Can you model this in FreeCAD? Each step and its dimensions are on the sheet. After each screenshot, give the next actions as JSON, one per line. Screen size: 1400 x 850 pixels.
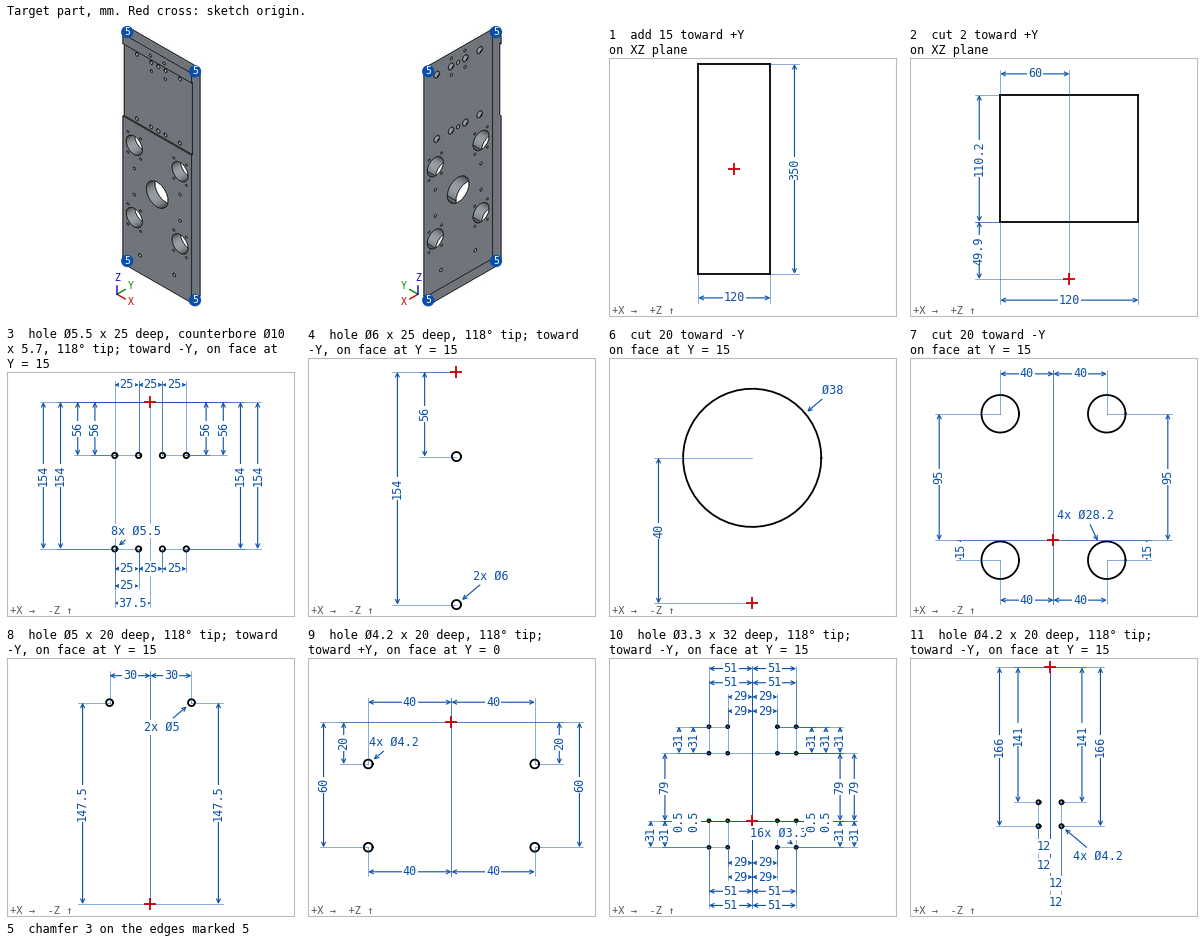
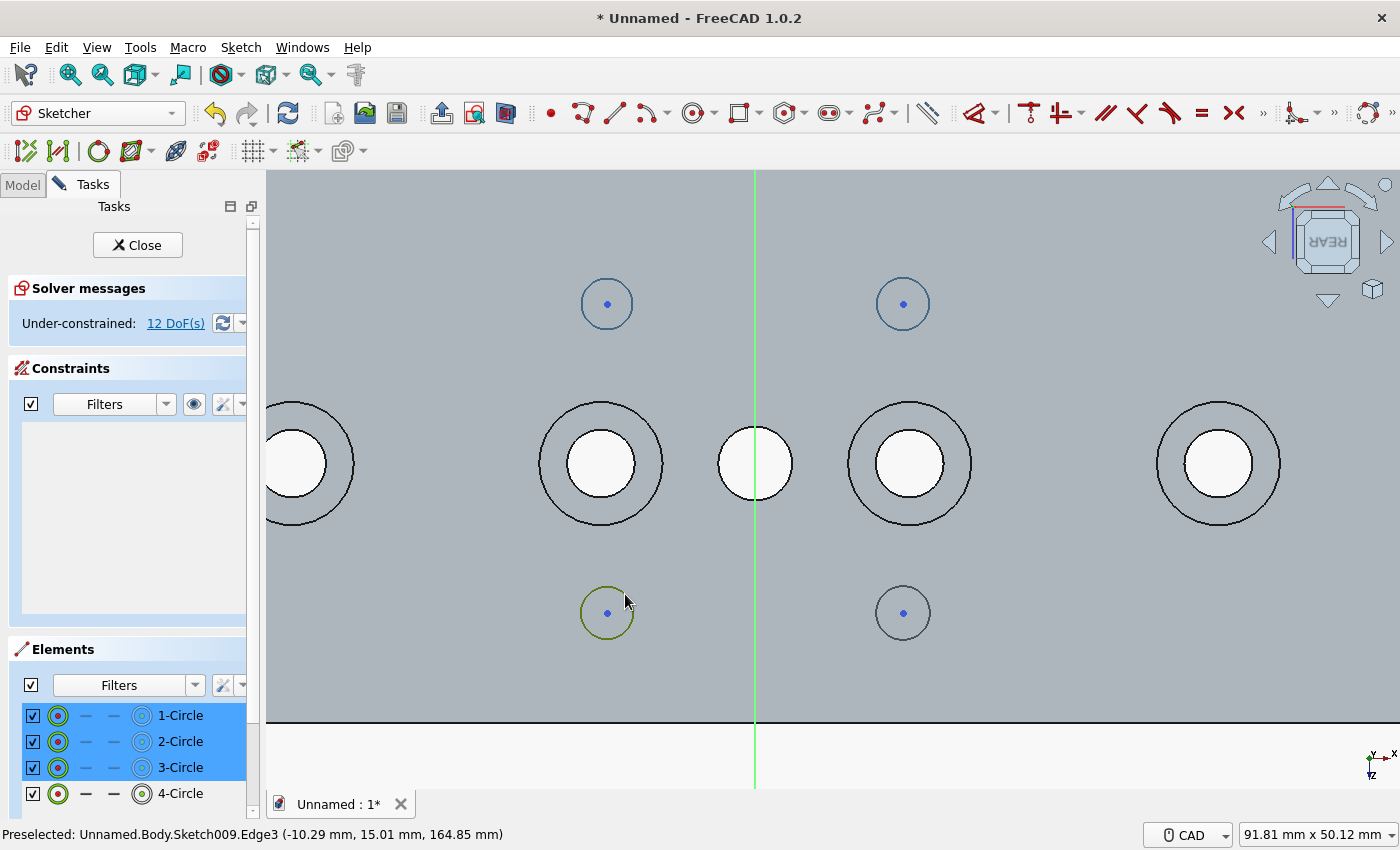
{"action": "left_click", "coordinate": [922, 594]}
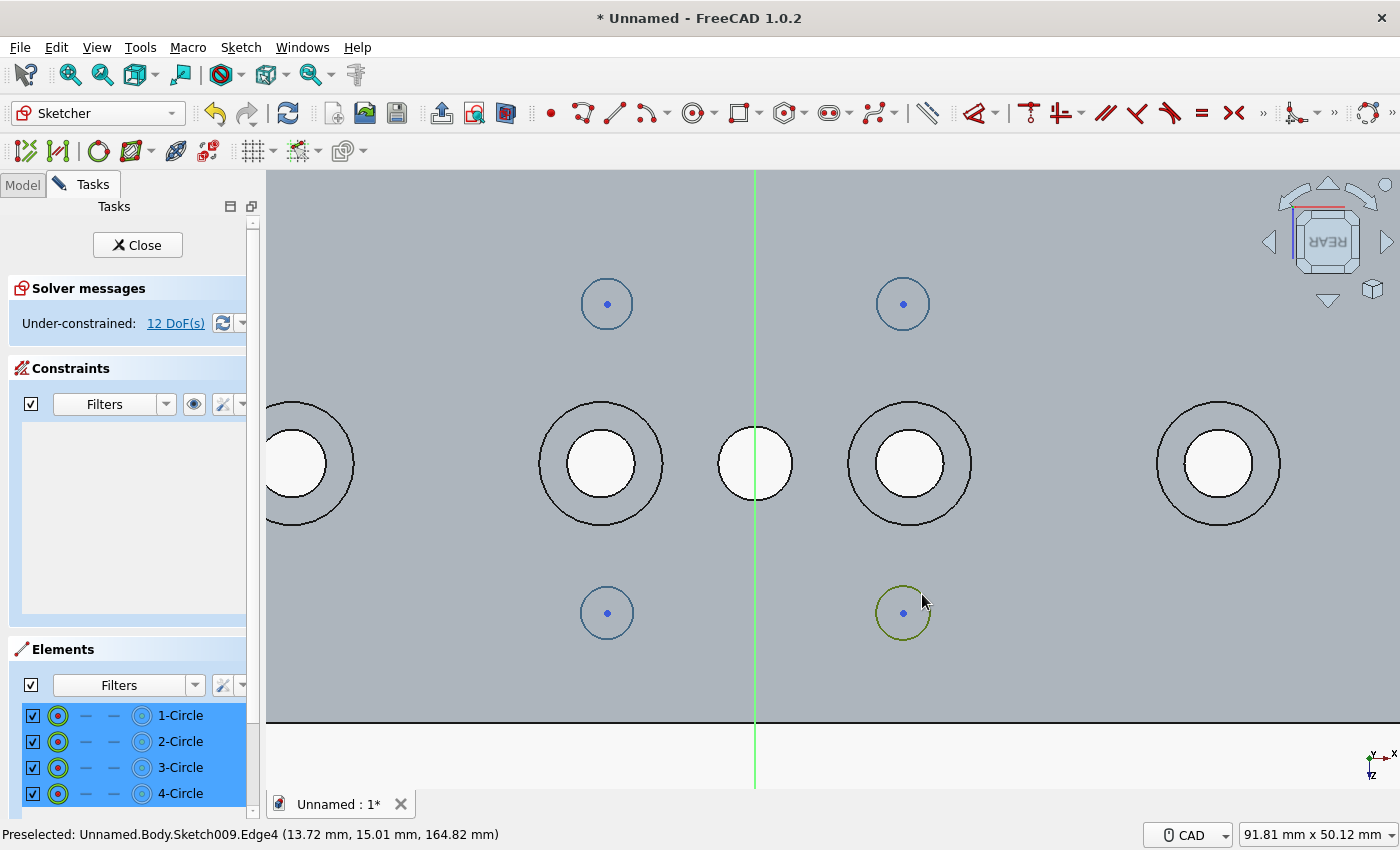
{"action": "left_click", "coordinate": [1202, 114]}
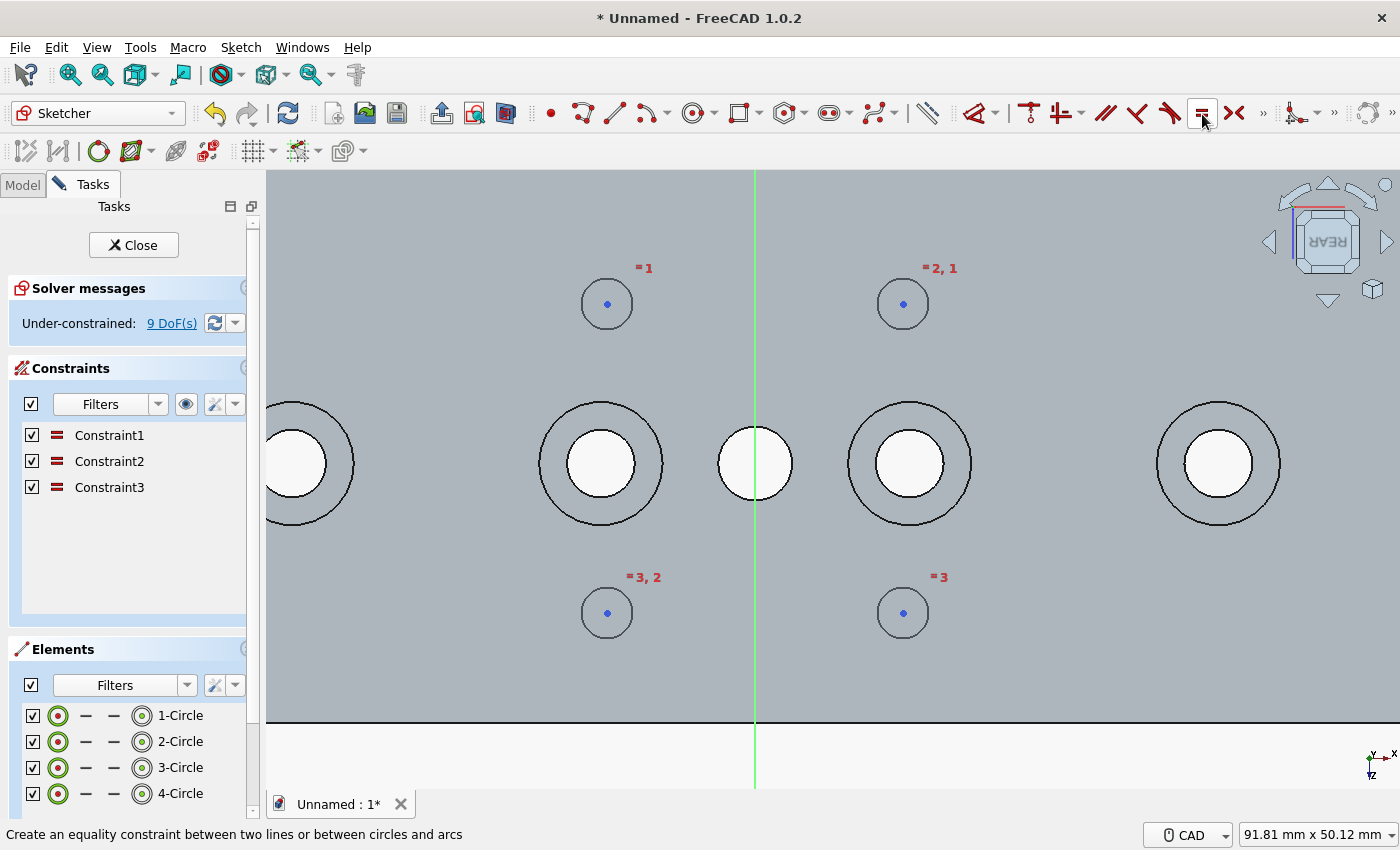
{"action": "left_click", "coordinate": [974, 114]}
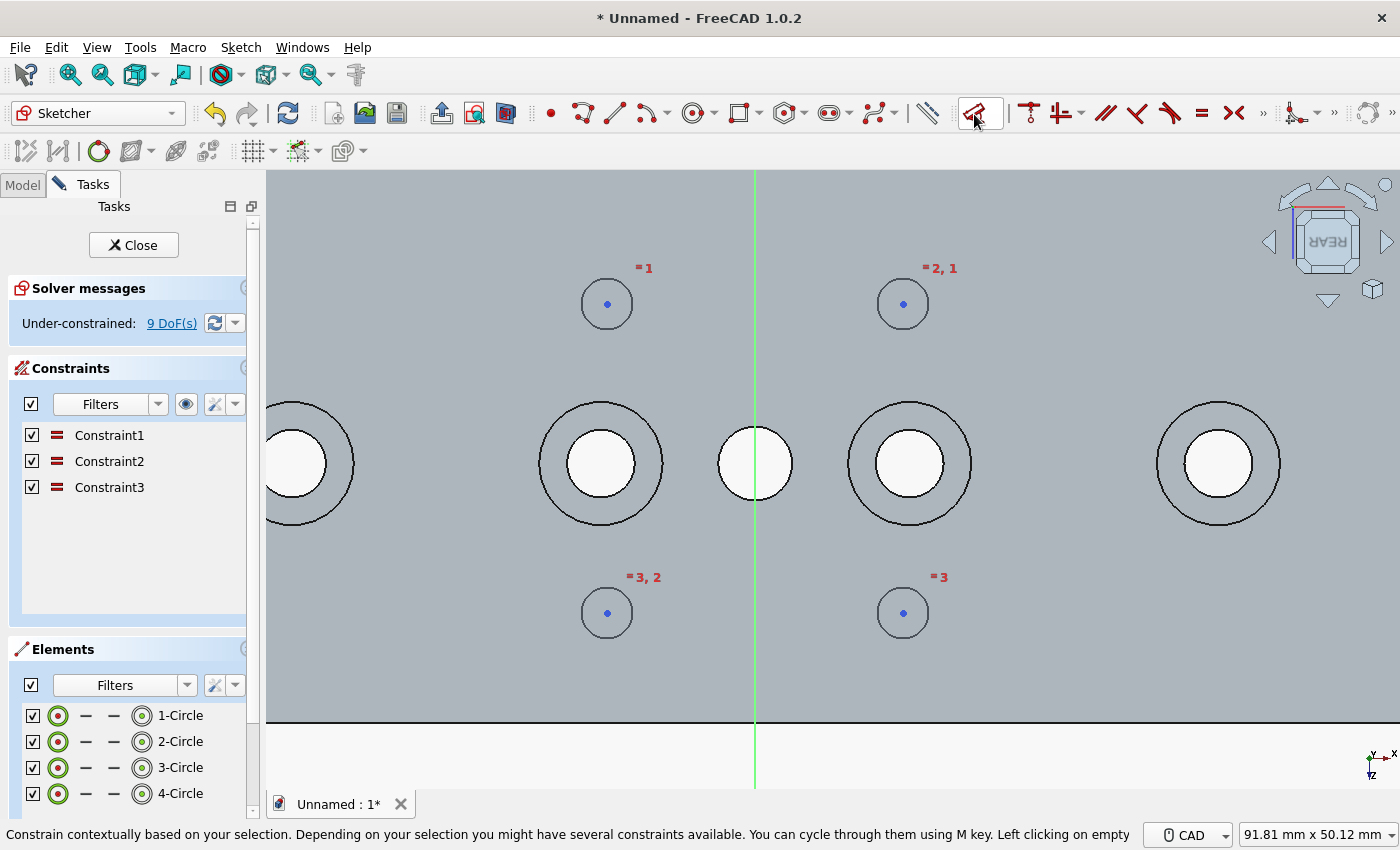
{"action": "left_click", "coordinate": [625, 286]}
{"action": "left_click", "coordinate": [648, 263]}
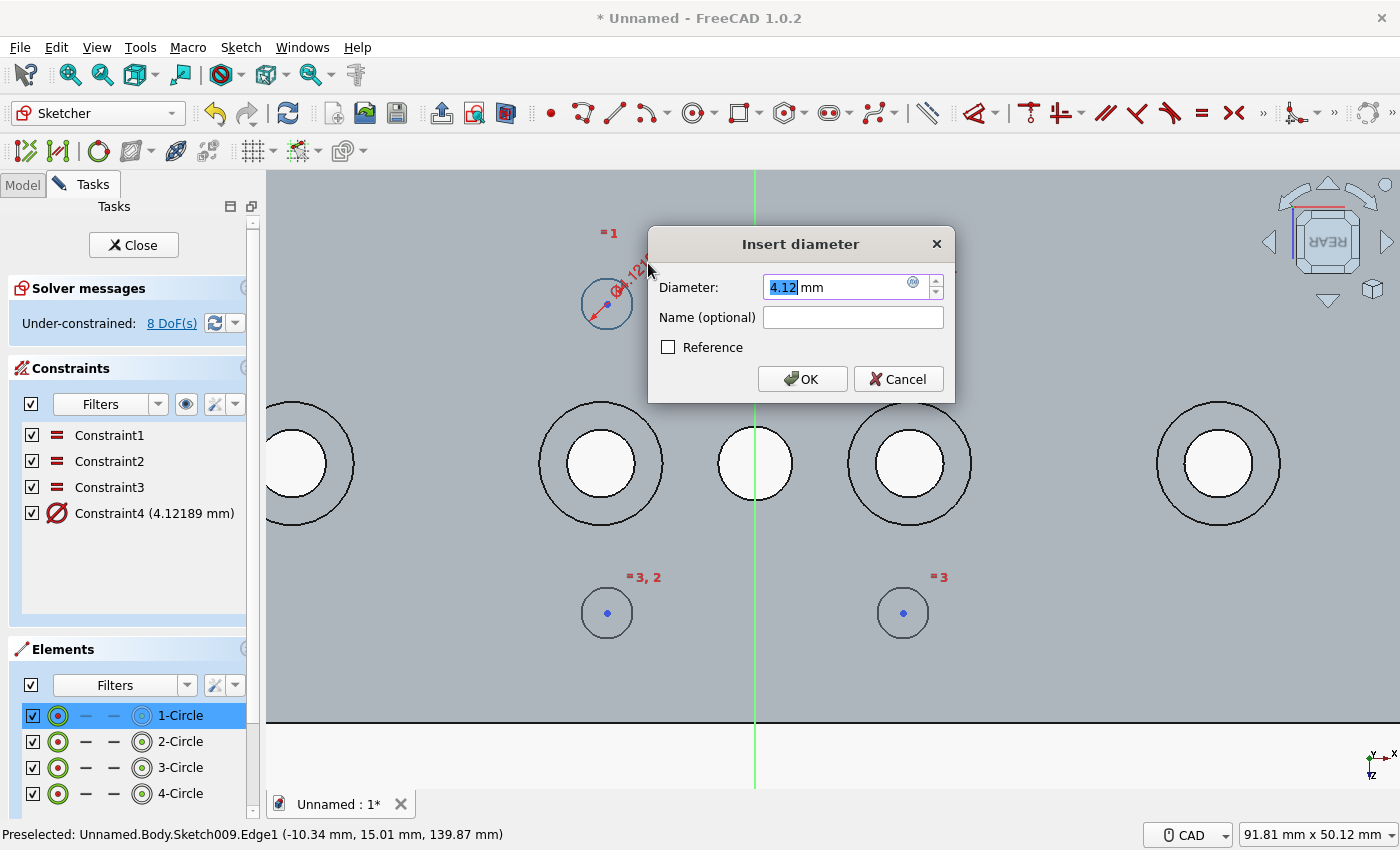
{"action": "type", "text": "4.2"}
{"action": "key", "text": "Return"}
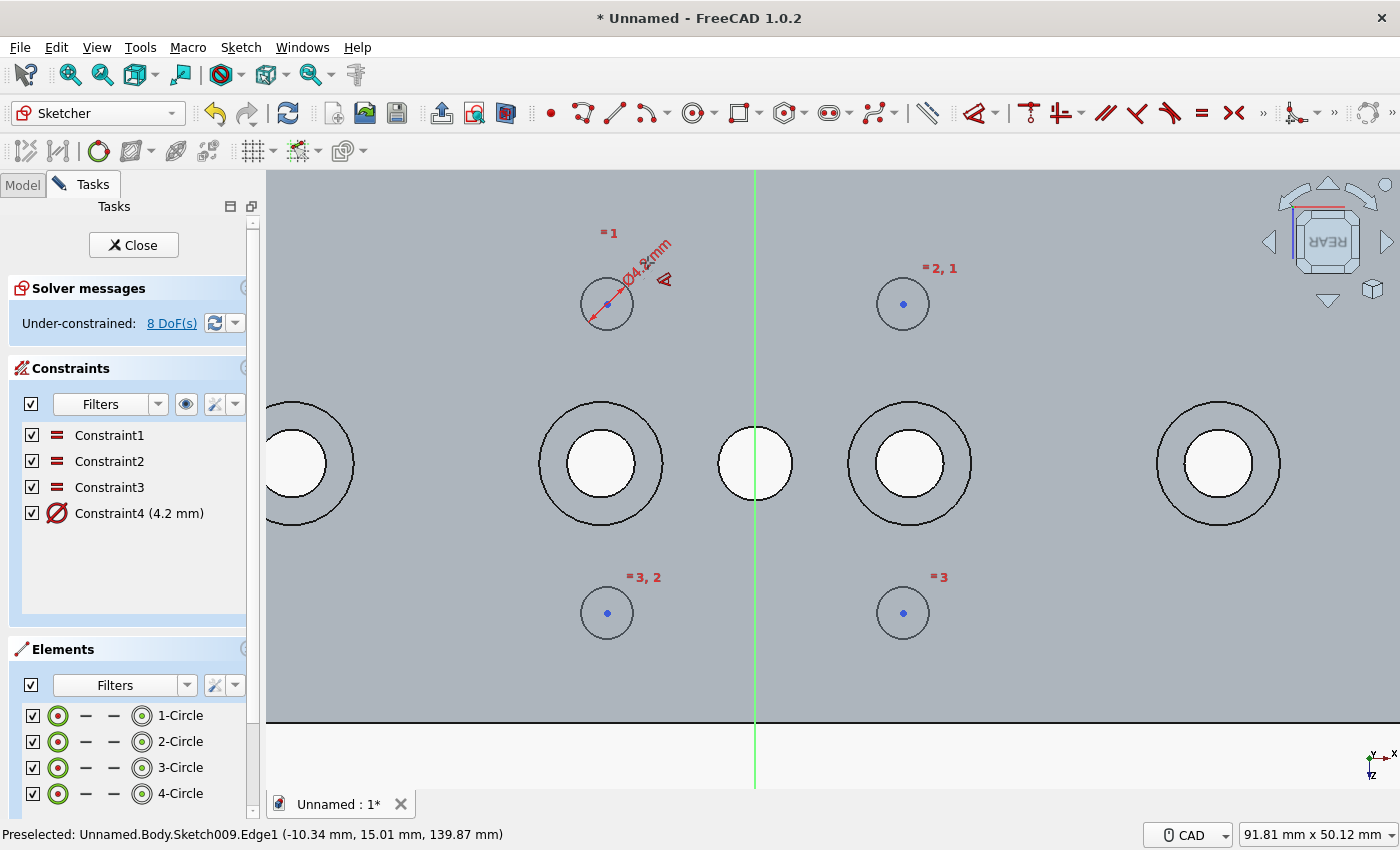
{"action": "left_click", "coordinate": [607, 304]}
{"action": "left_click", "coordinate": [681, 338]}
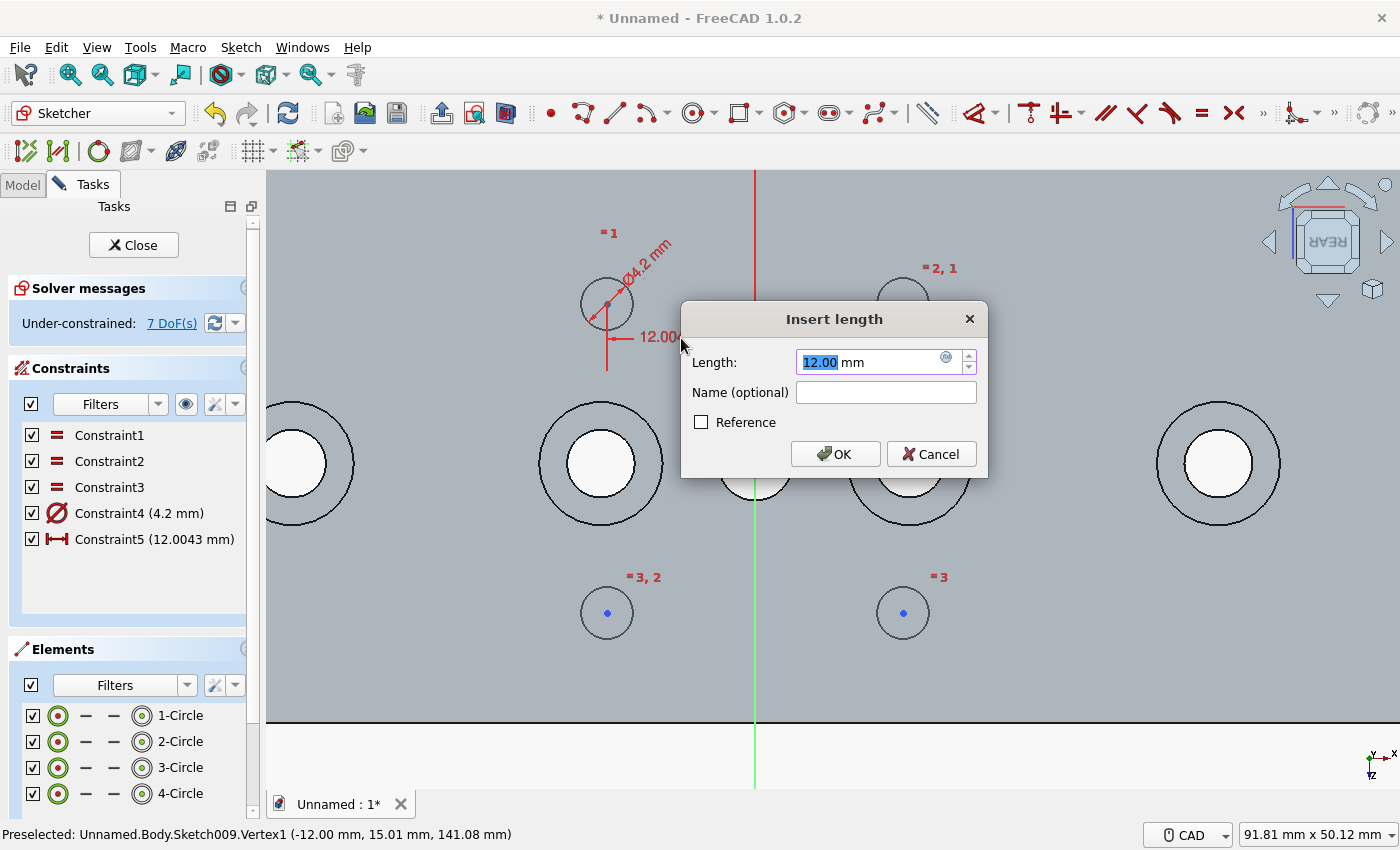
{"action": "type", "text": "12"}
{"action": "key", "text": "Return"}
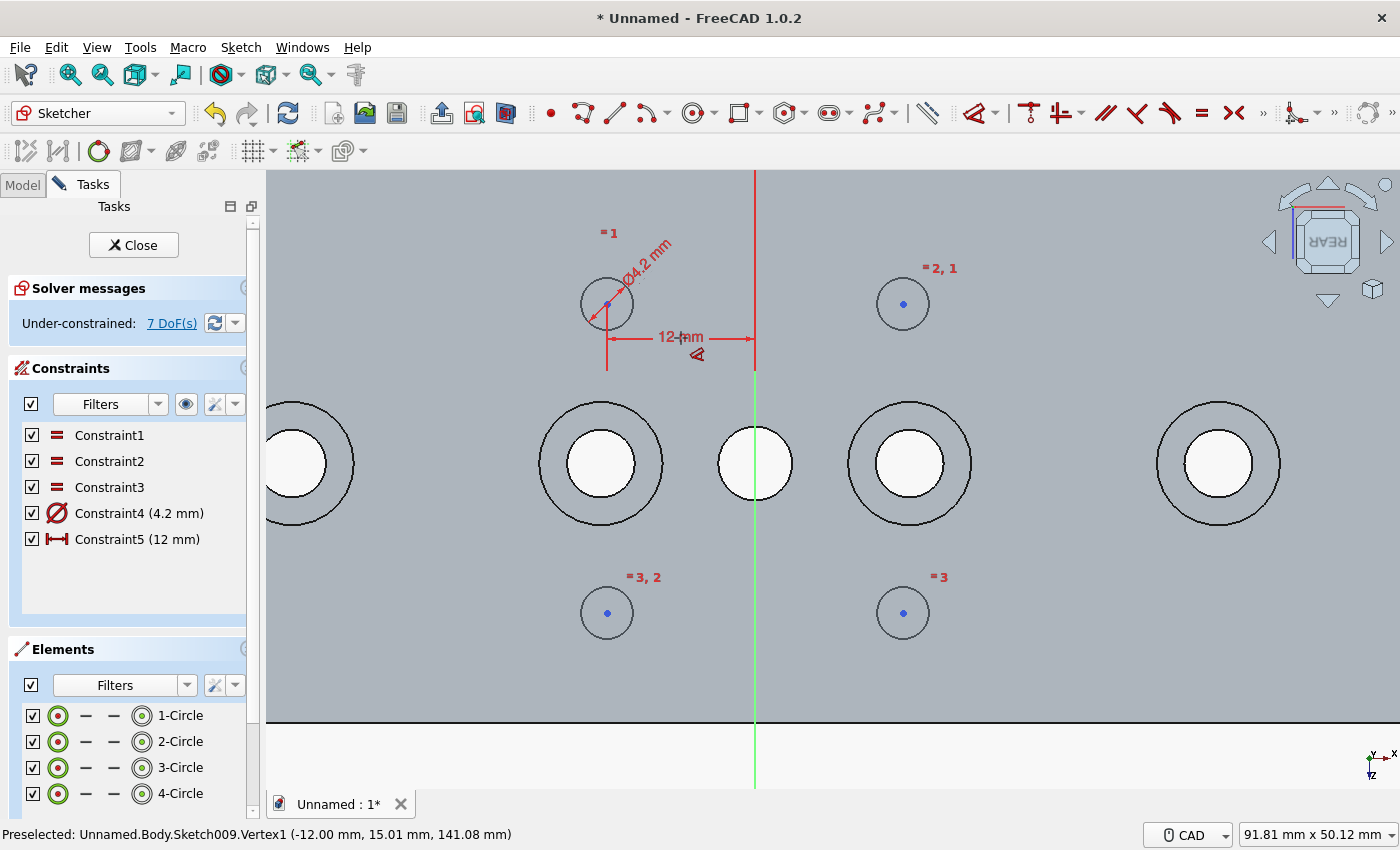
{"action": "left_click", "coordinate": [903, 304]}
{"action": "left_click", "coordinate": [829, 338]}